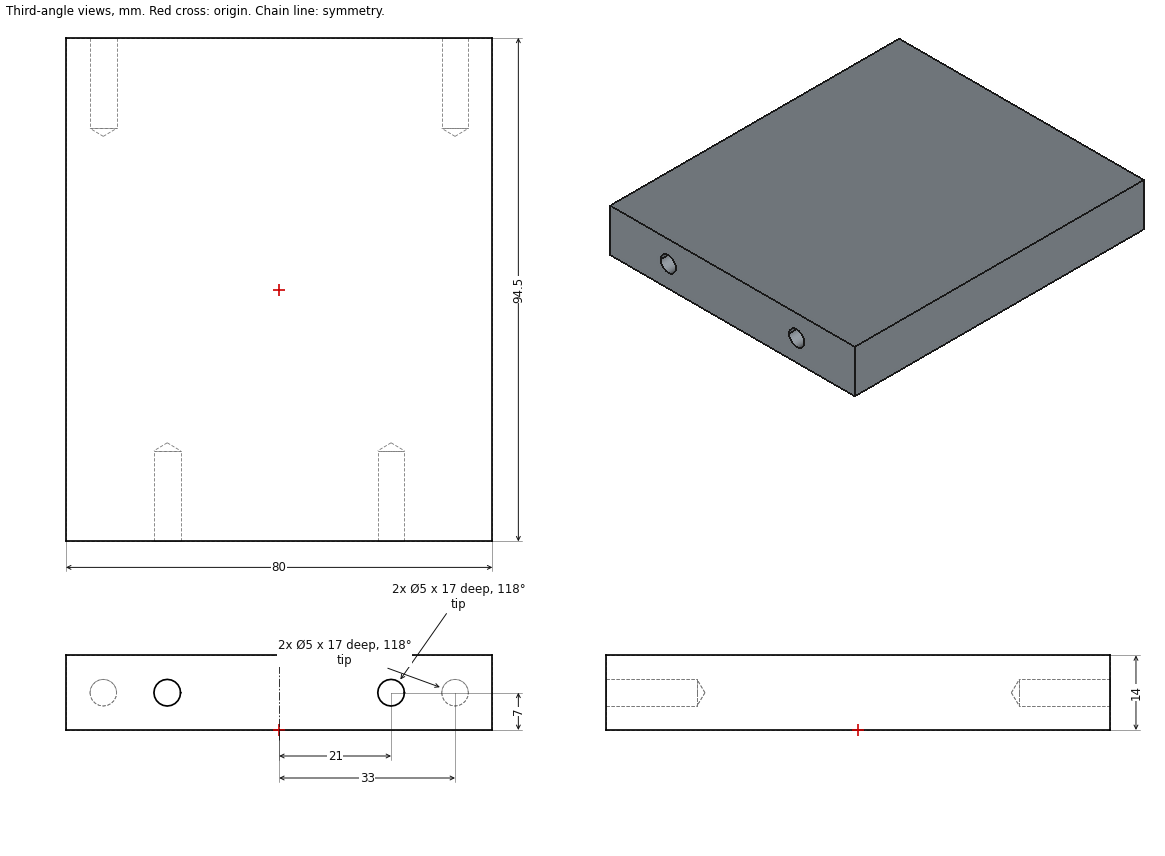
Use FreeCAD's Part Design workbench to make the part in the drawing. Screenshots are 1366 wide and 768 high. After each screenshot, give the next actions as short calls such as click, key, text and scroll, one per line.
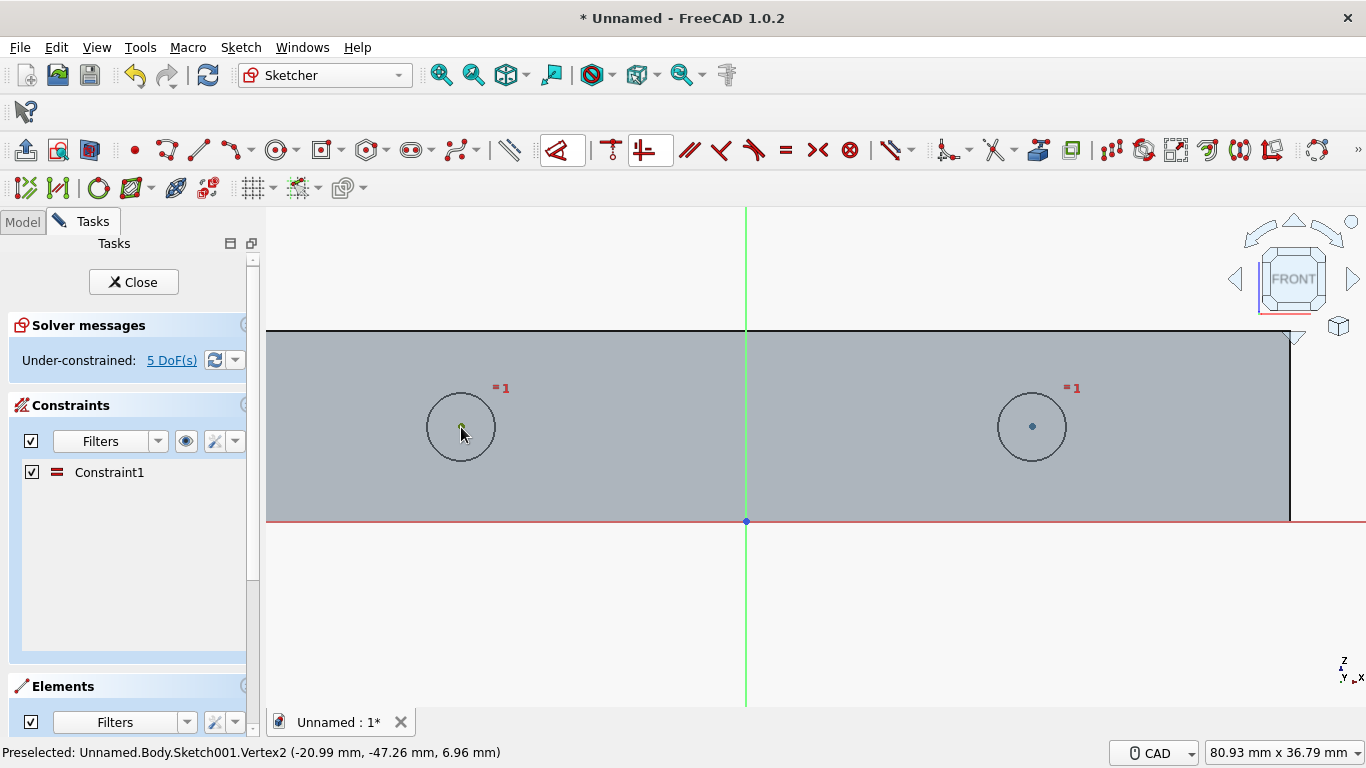
click(746, 647)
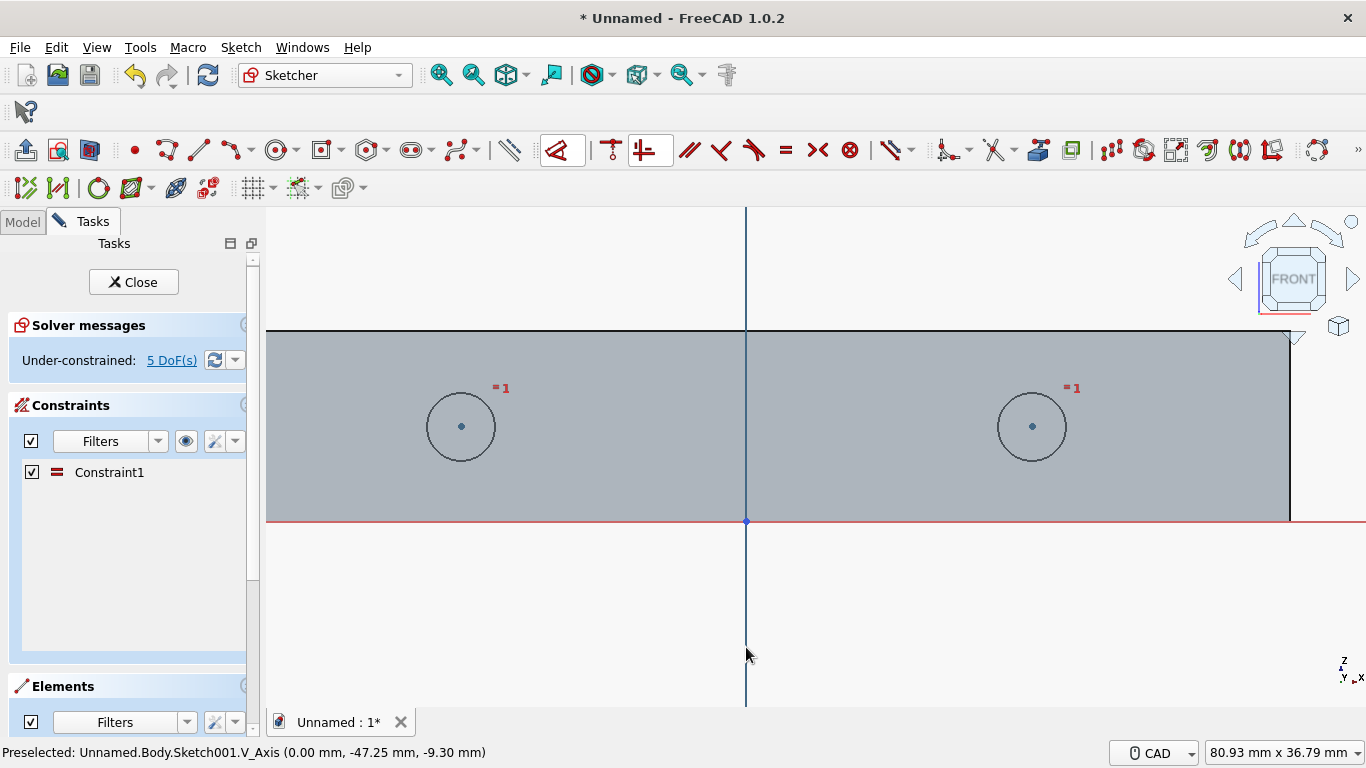
key(s)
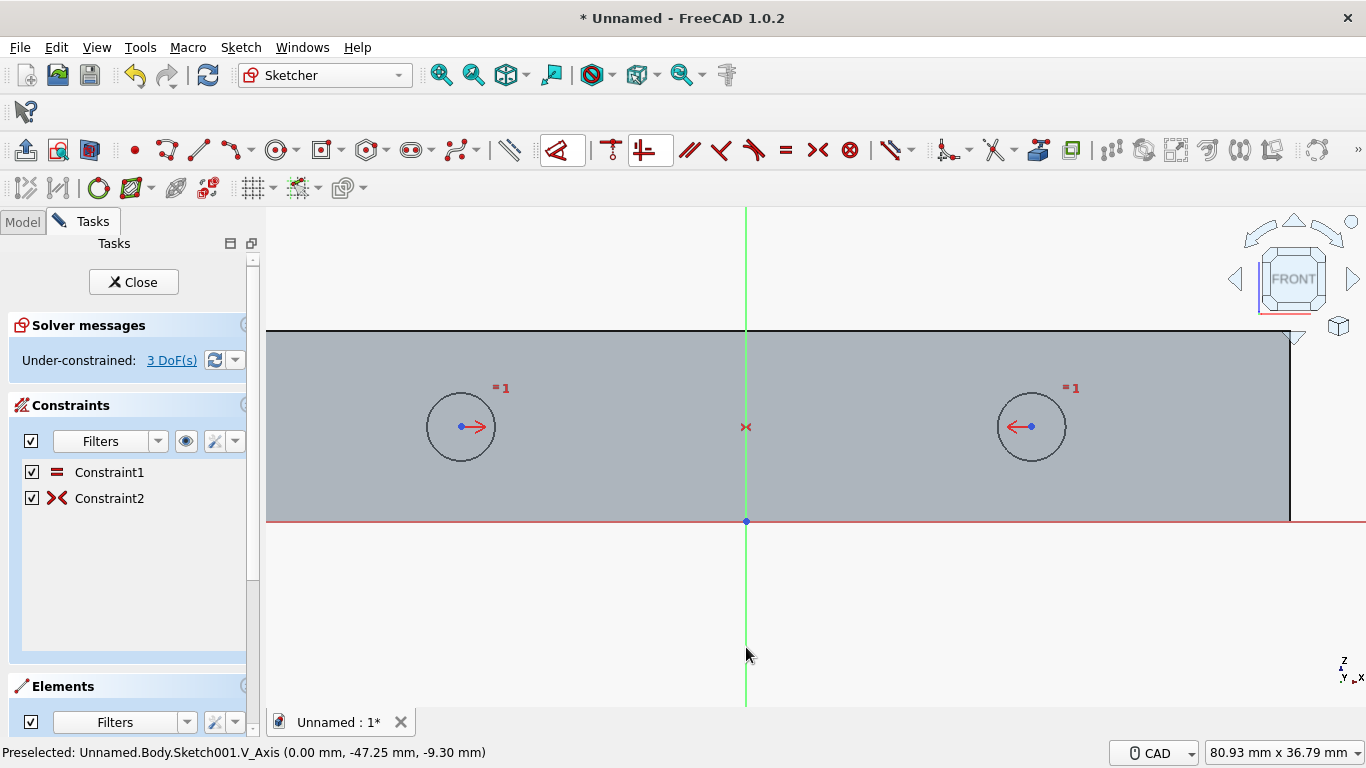
click(556, 150)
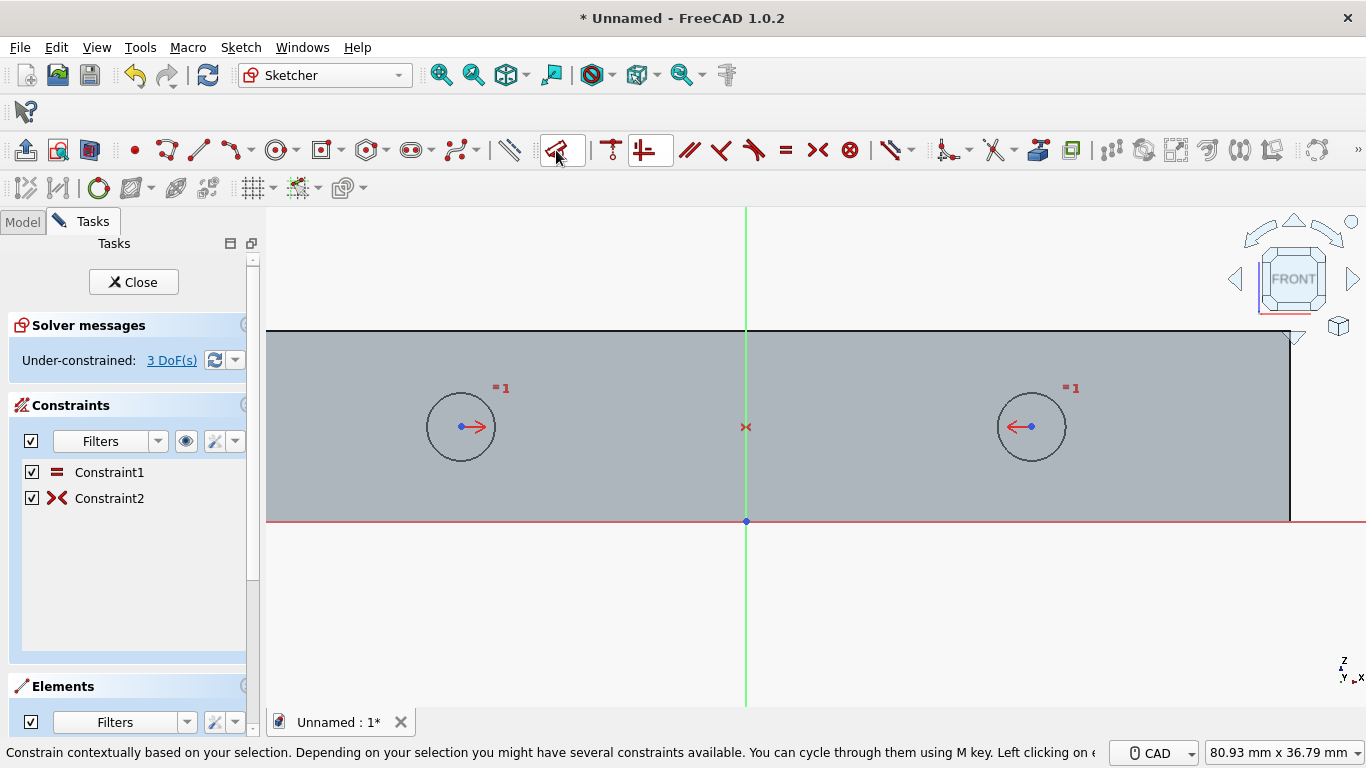
click(1056, 403)
click(1079, 381)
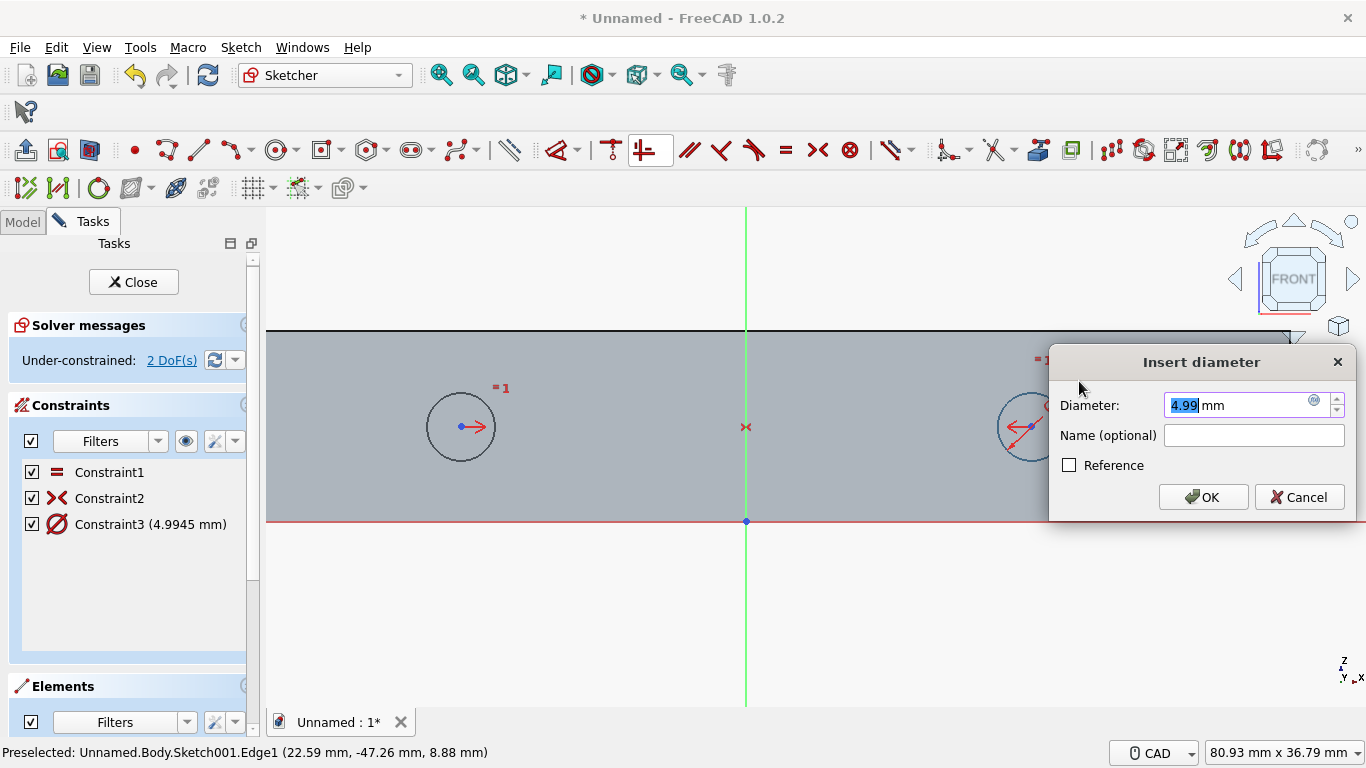
text(5)
key(Return)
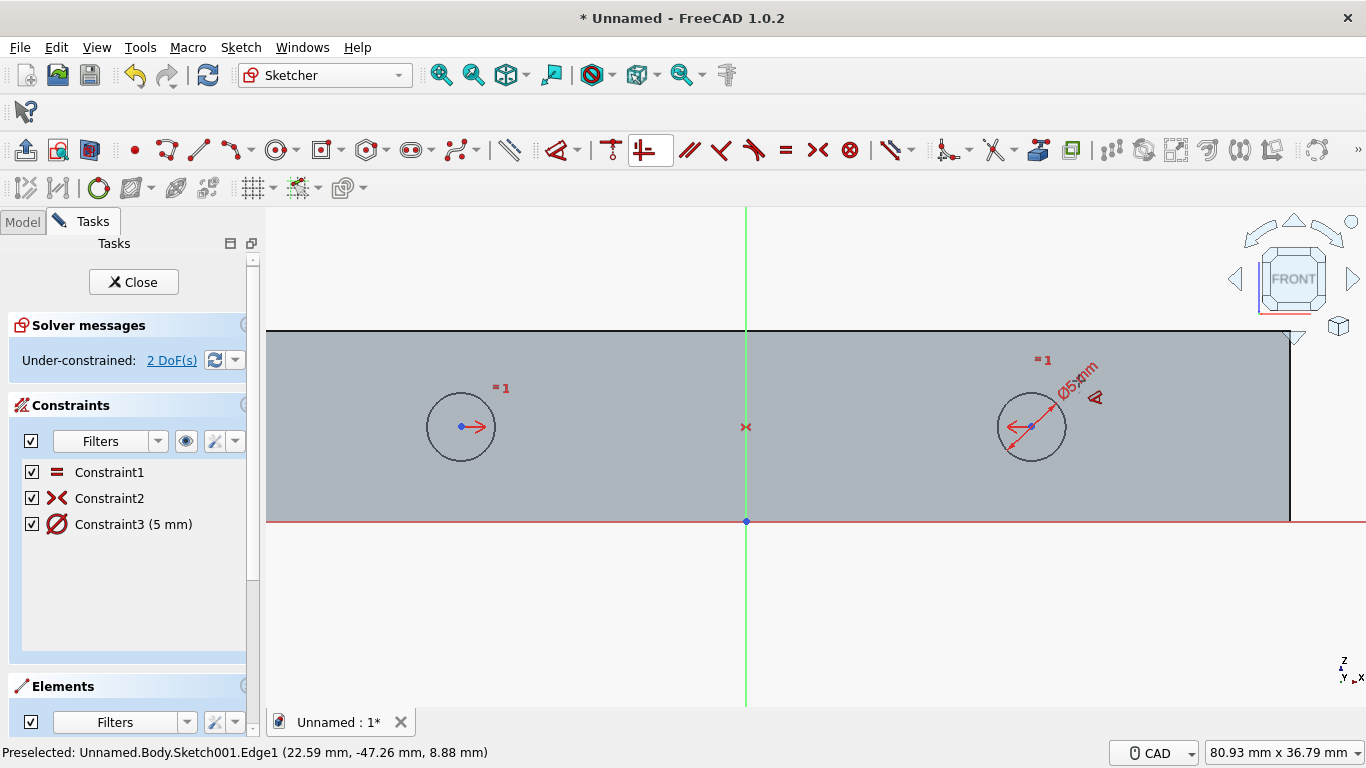
click(1032, 427)
click(1066, 474)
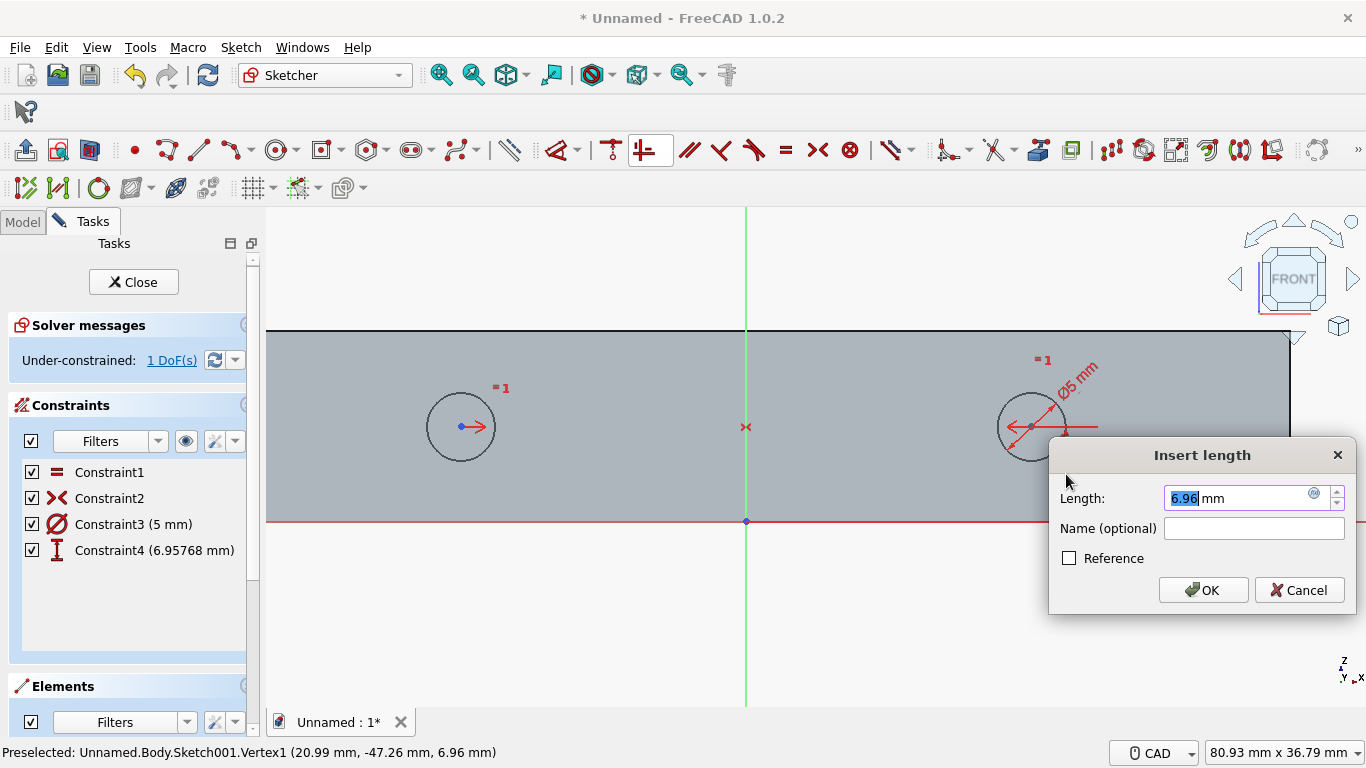
text(7)
key(Return)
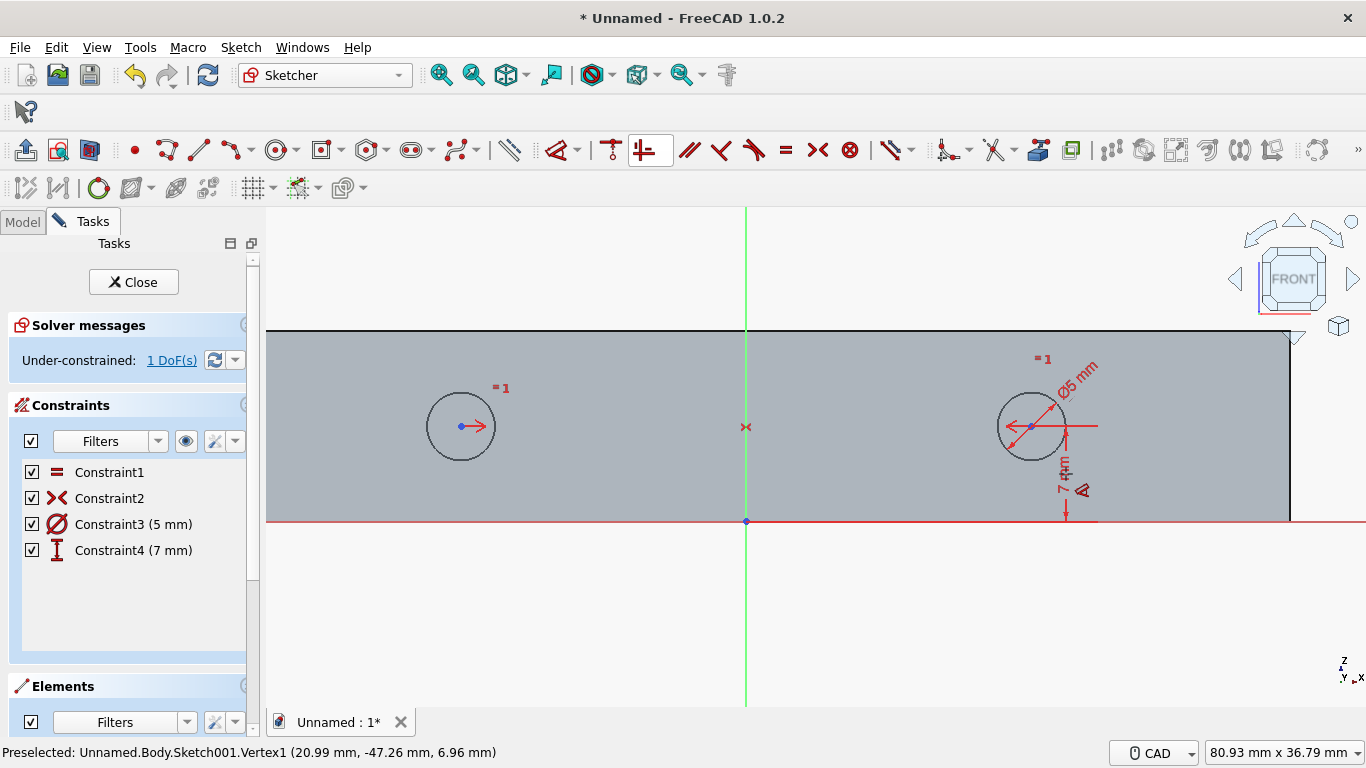
click(1032, 426)
click(889, 556)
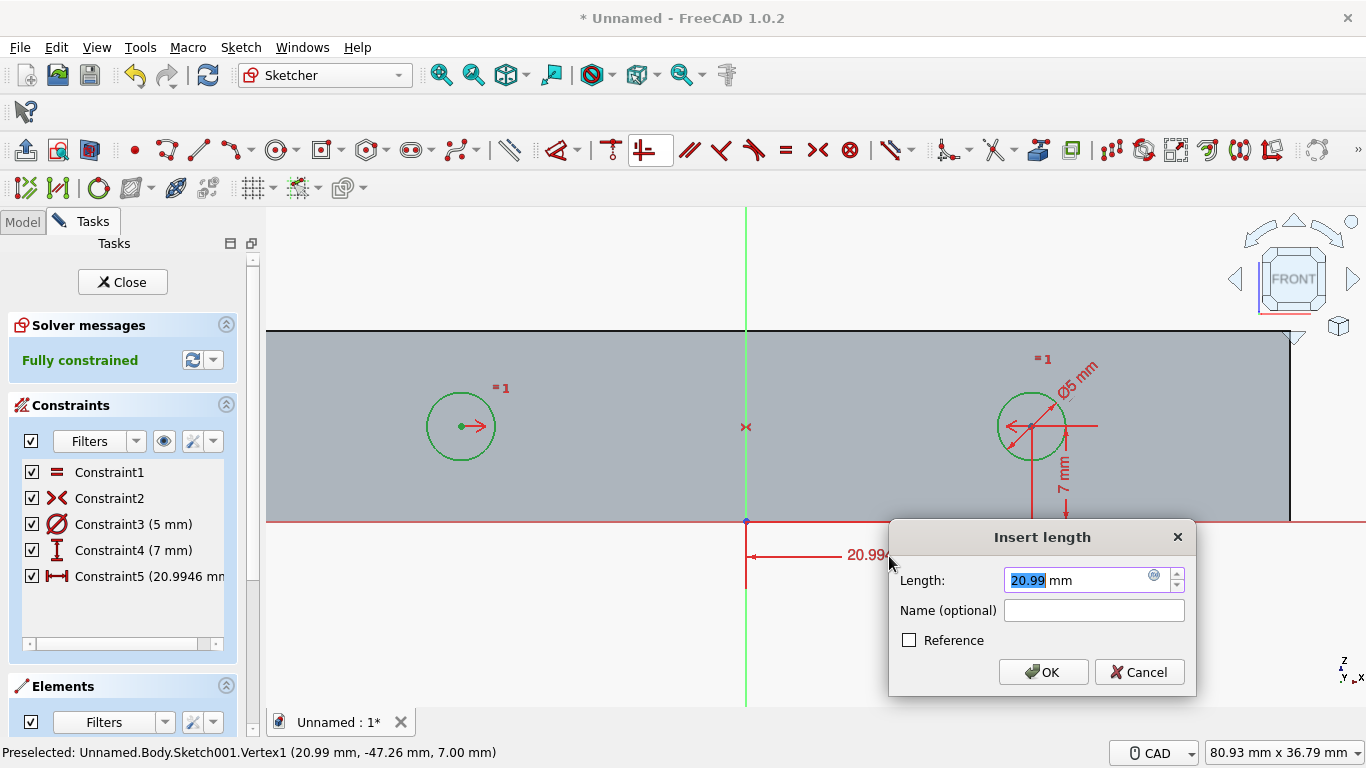
text(21)
key(Return)
key(Escape)